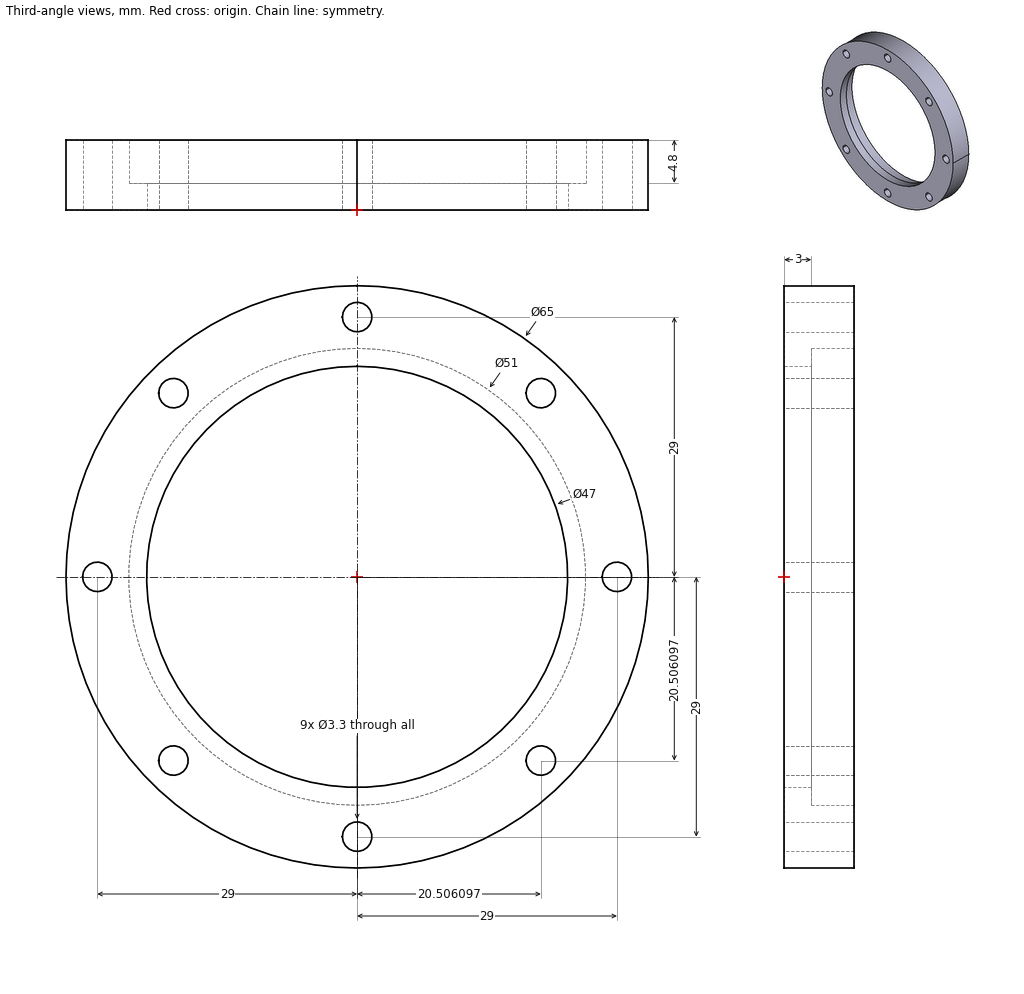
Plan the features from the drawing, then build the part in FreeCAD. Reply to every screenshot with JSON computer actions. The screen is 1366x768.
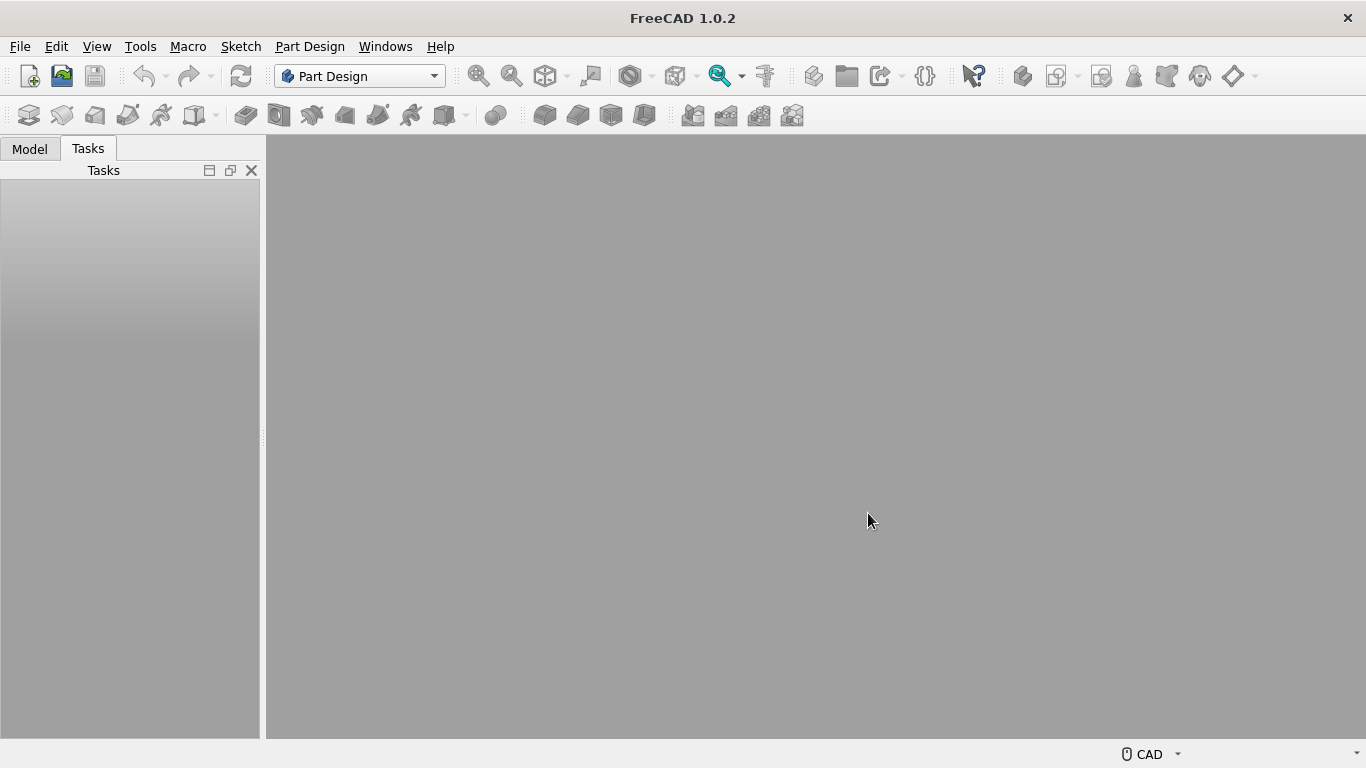
{"action": "left_click", "coordinate": [29, 76]}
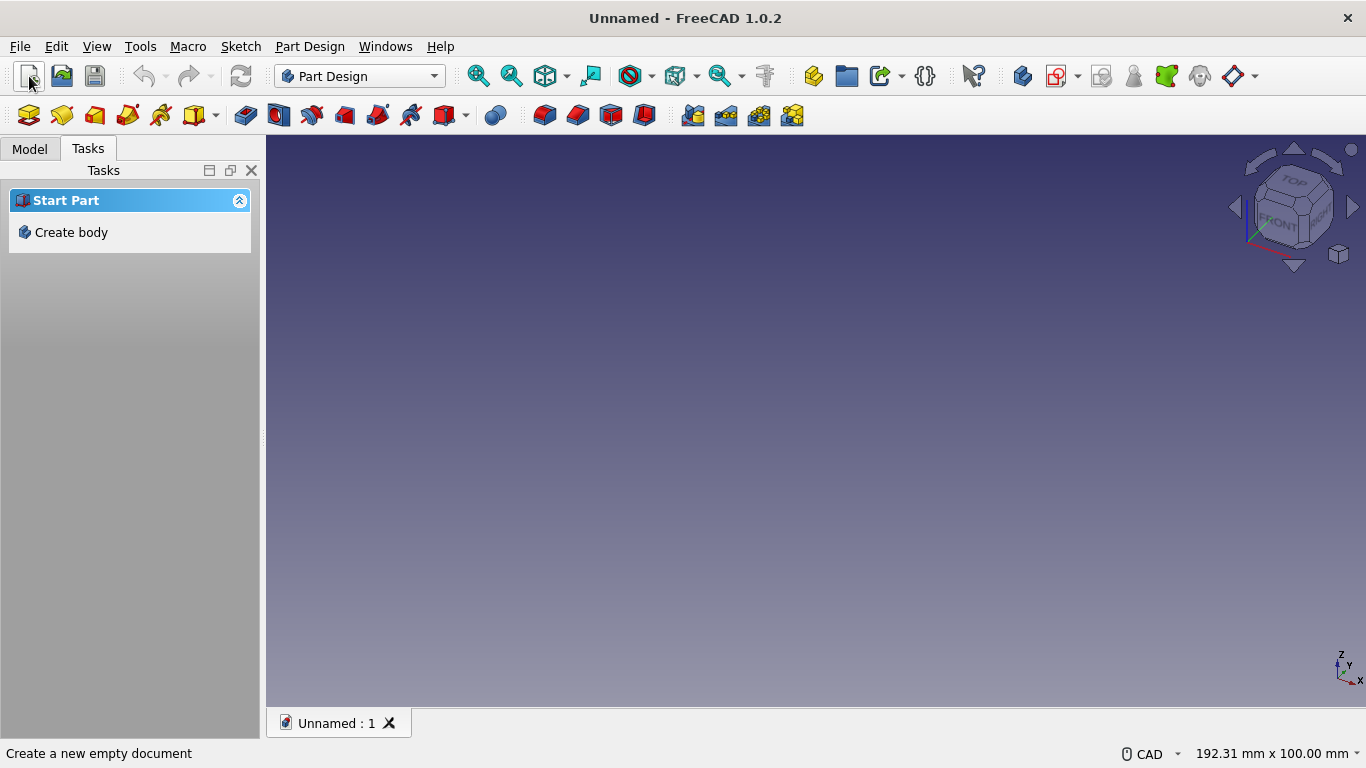
{"action": "left_click", "coordinate": [1056, 76]}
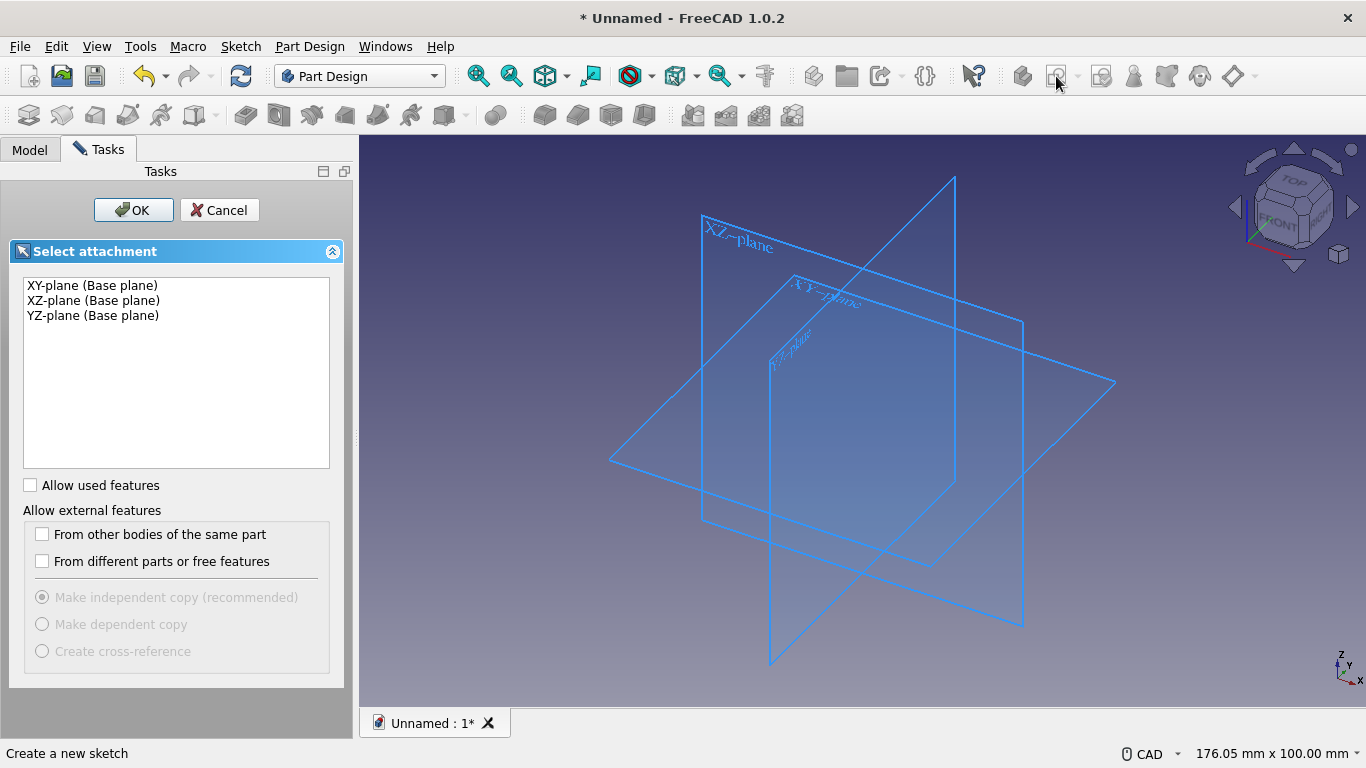
{"action": "left_click", "coordinate": [84, 300]}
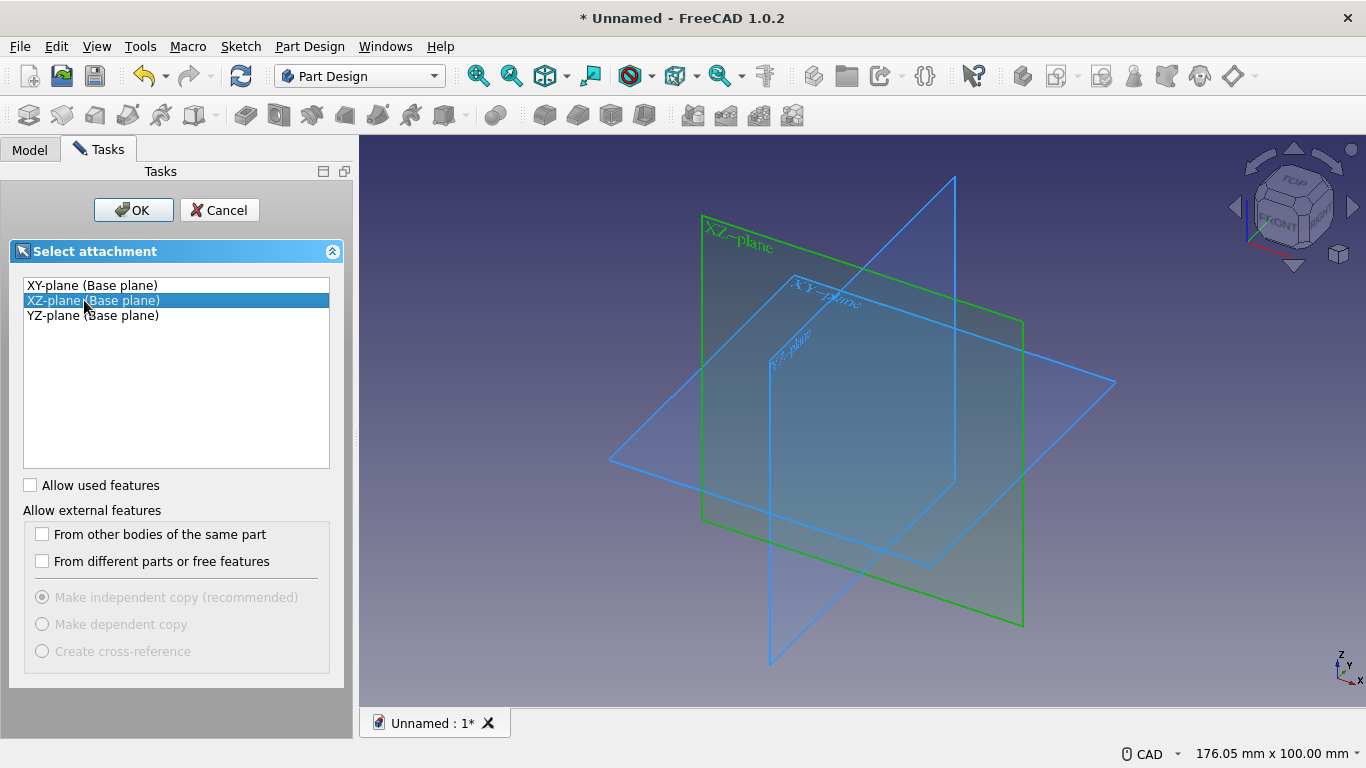
{"action": "left_click", "coordinate": [134, 210]}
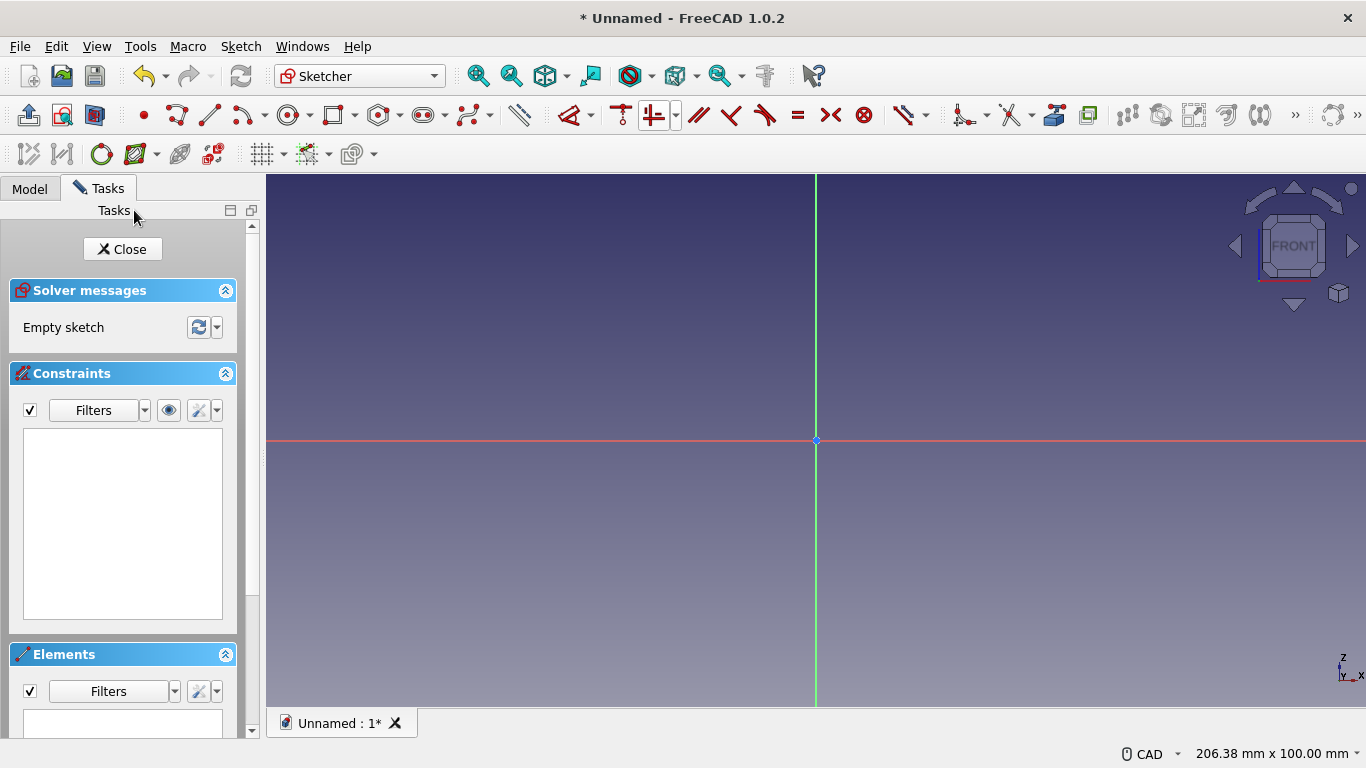
{"action": "left_click", "coordinate": [288, 116]}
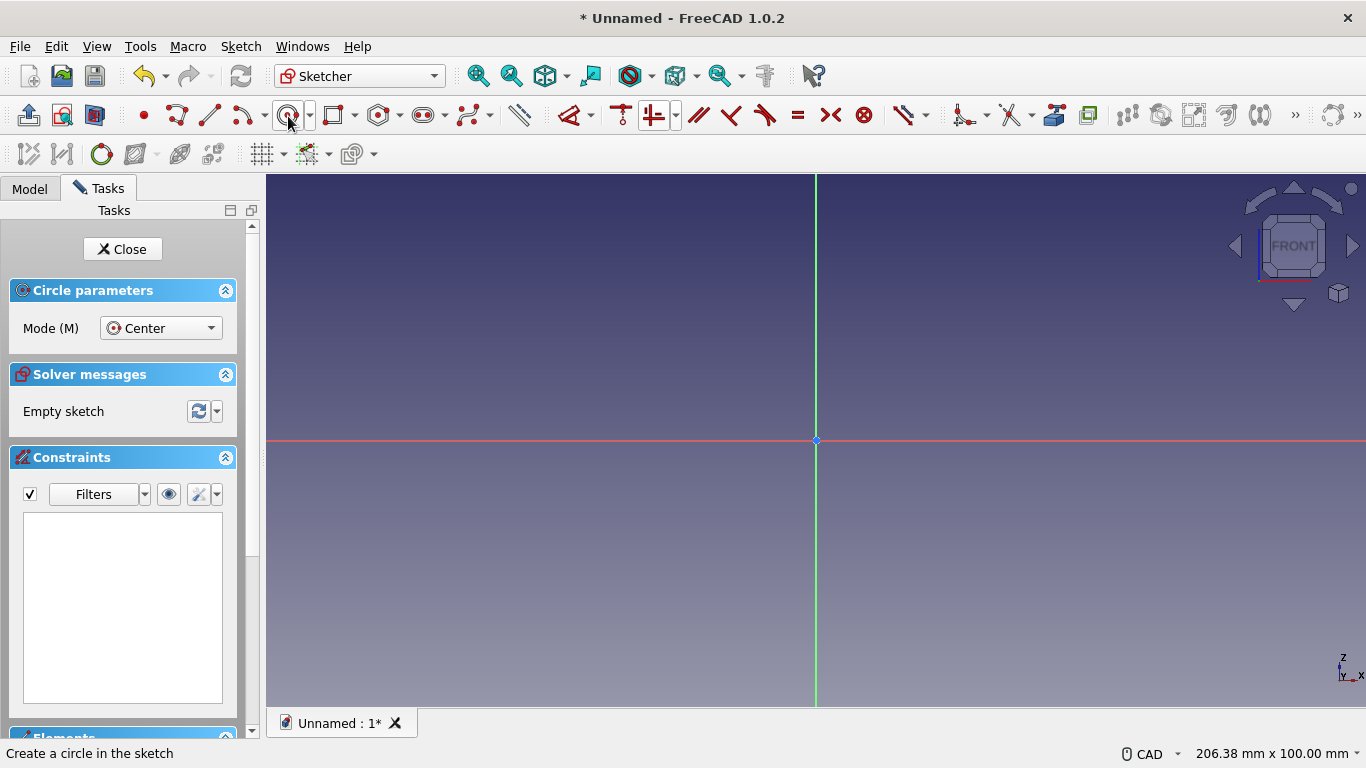
{"action": "left_click", "coordinate": [816, 440]}
{"action": "mouse_move", "coordinate": [938, 318]}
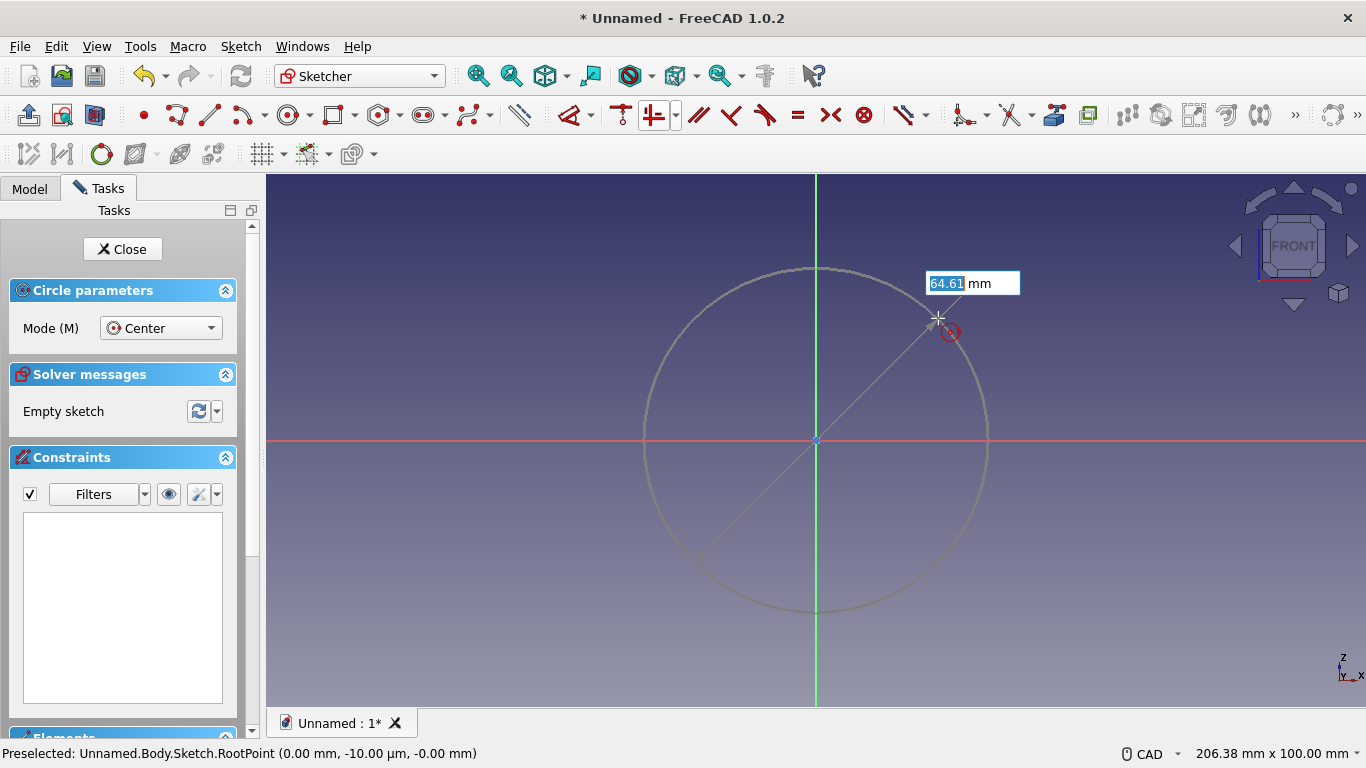
{"action": "type", "text": "65"}
{"action": "key", "text": "Return"}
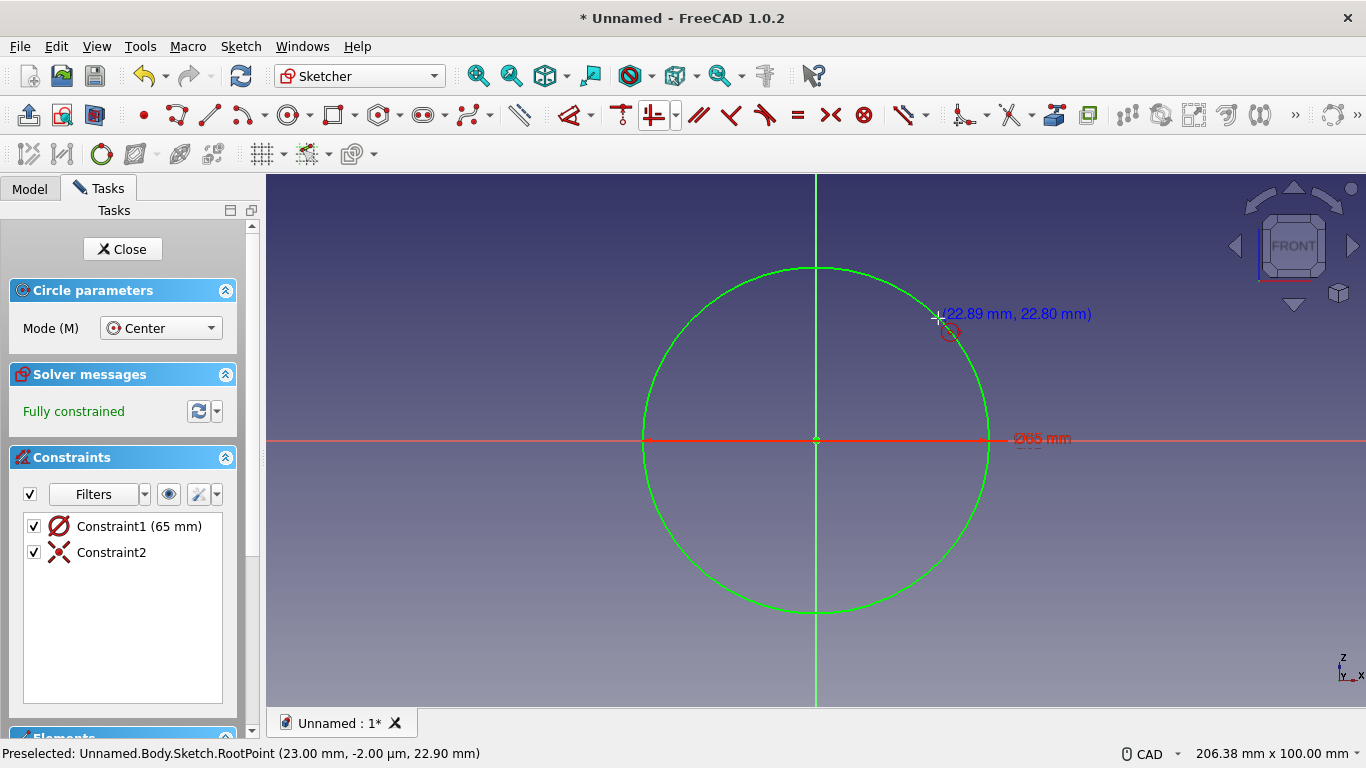
{"action": "left_click", "coordinate": [816, 440]}
{"action": "mouse_move", "coordinate": [905, 352]}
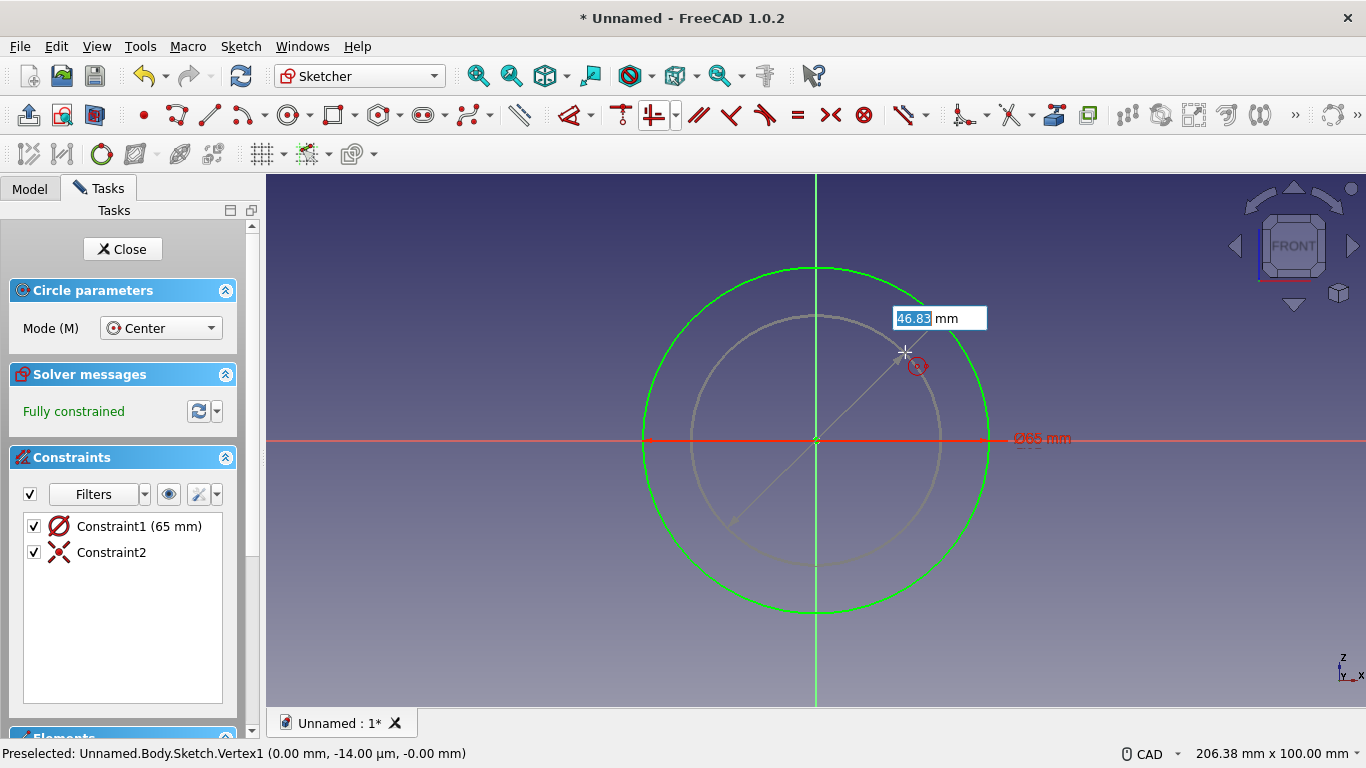
{"action": "type", "text": "47"}
{"action": "key", "text": "Return"}
{"action": "key", "text": "Escape"}